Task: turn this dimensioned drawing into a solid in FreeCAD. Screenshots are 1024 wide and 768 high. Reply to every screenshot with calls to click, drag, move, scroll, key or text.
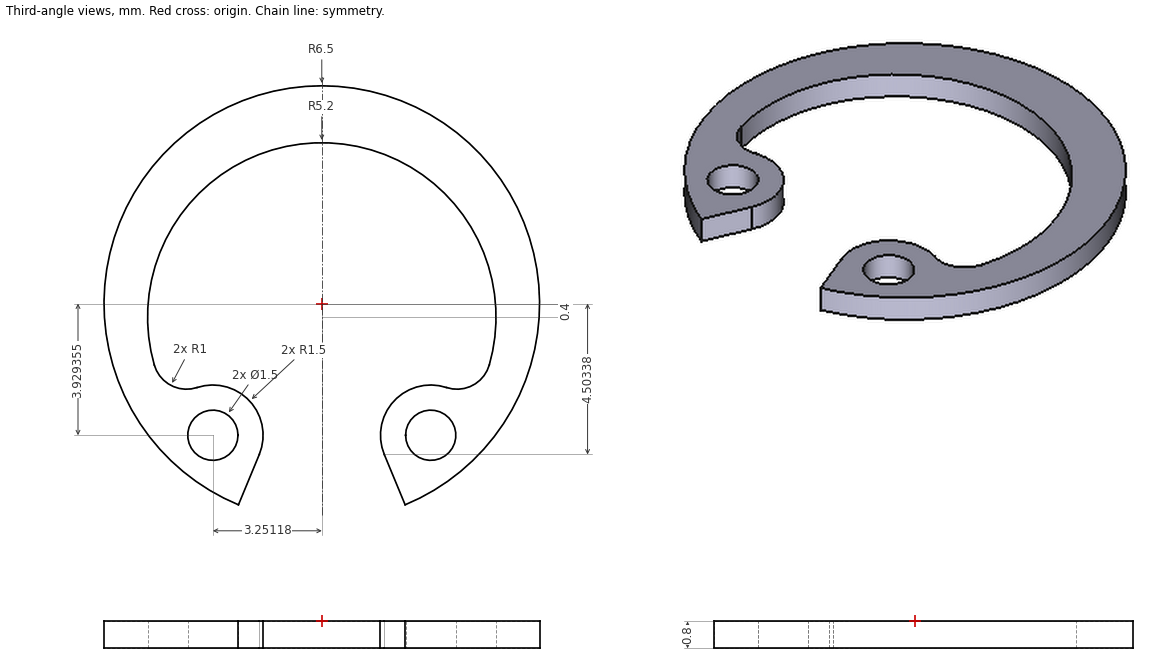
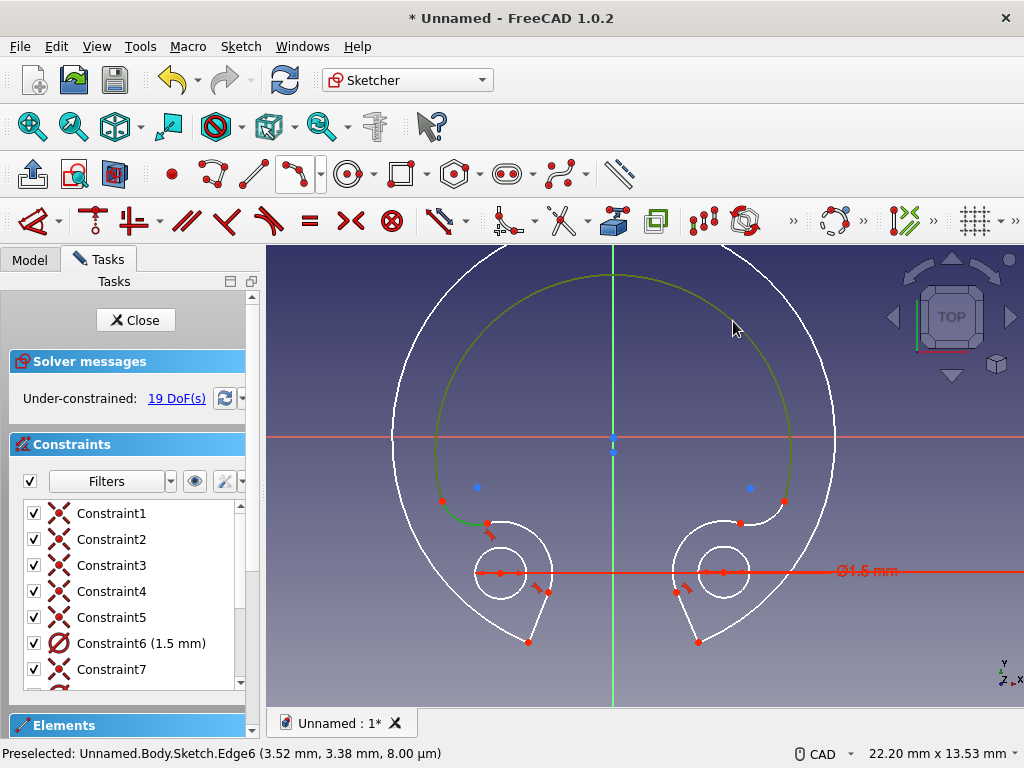
key(t)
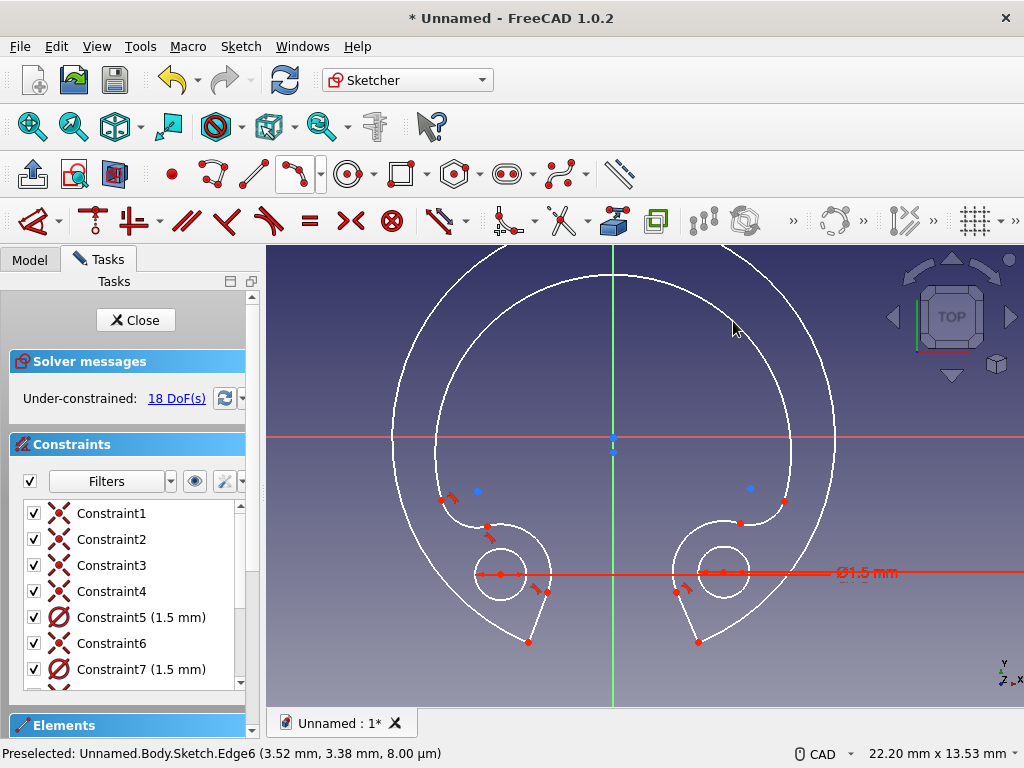
click(733, 321)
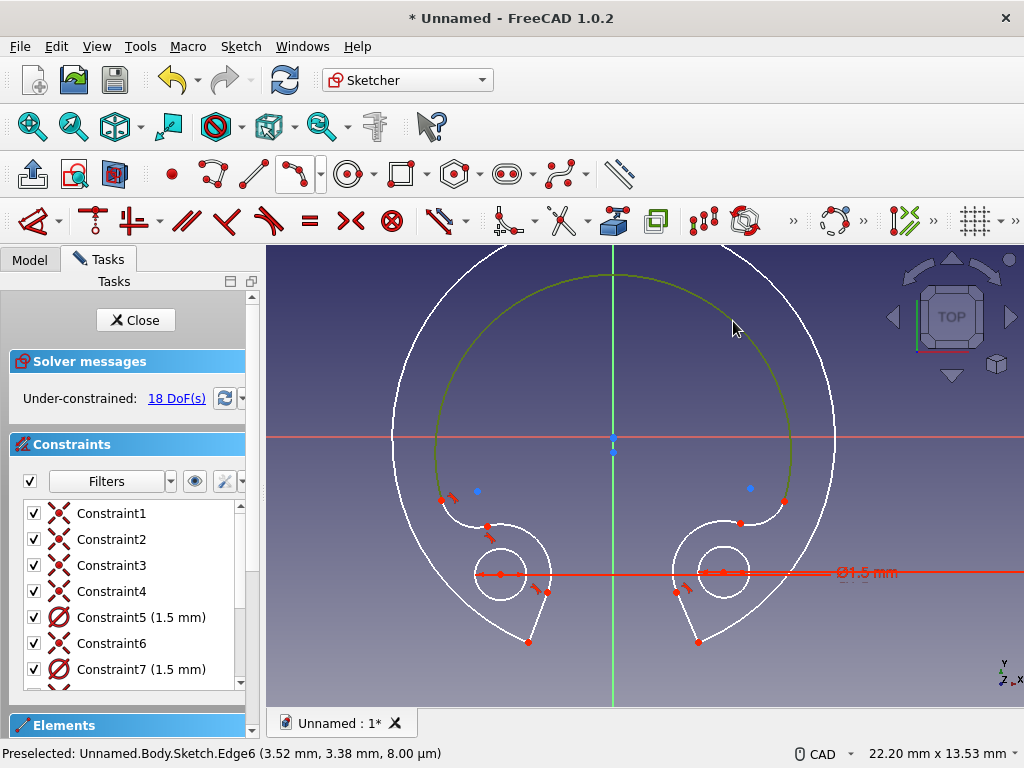
click(757, 524)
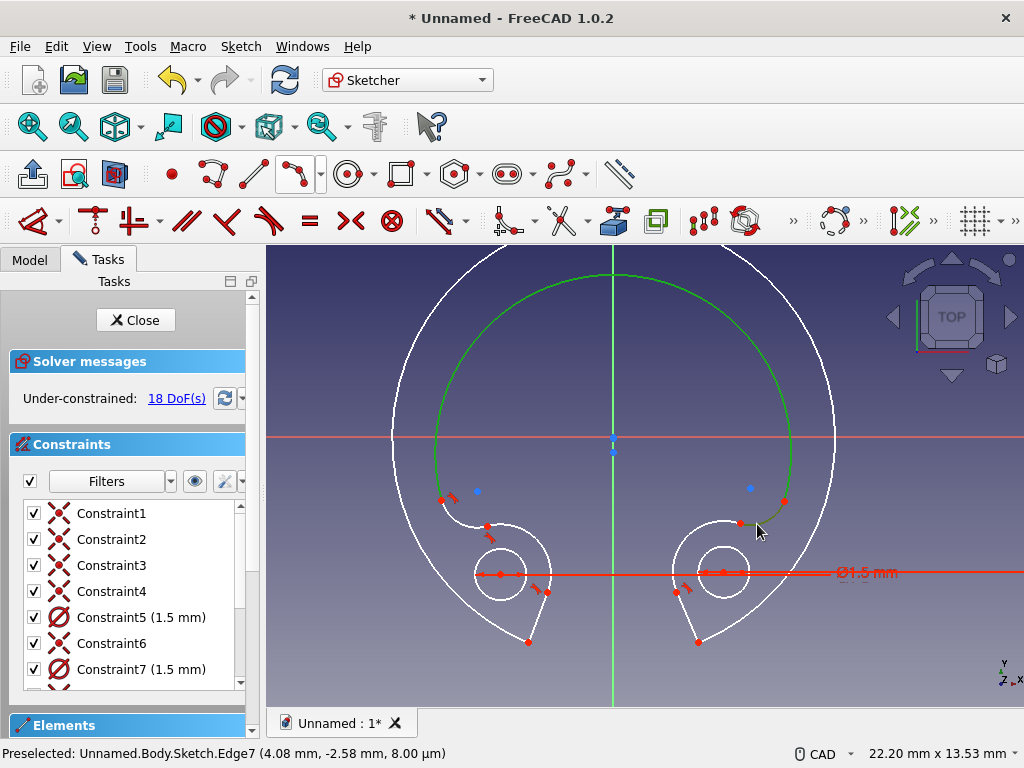
click(269, 222)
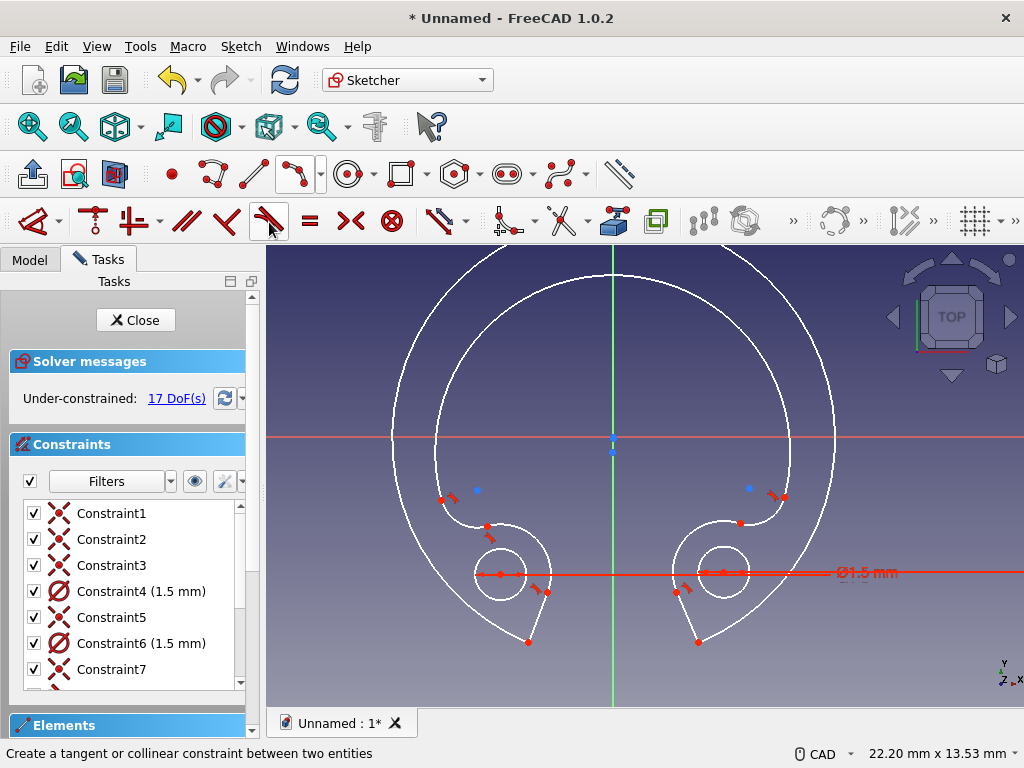
click(758, 524)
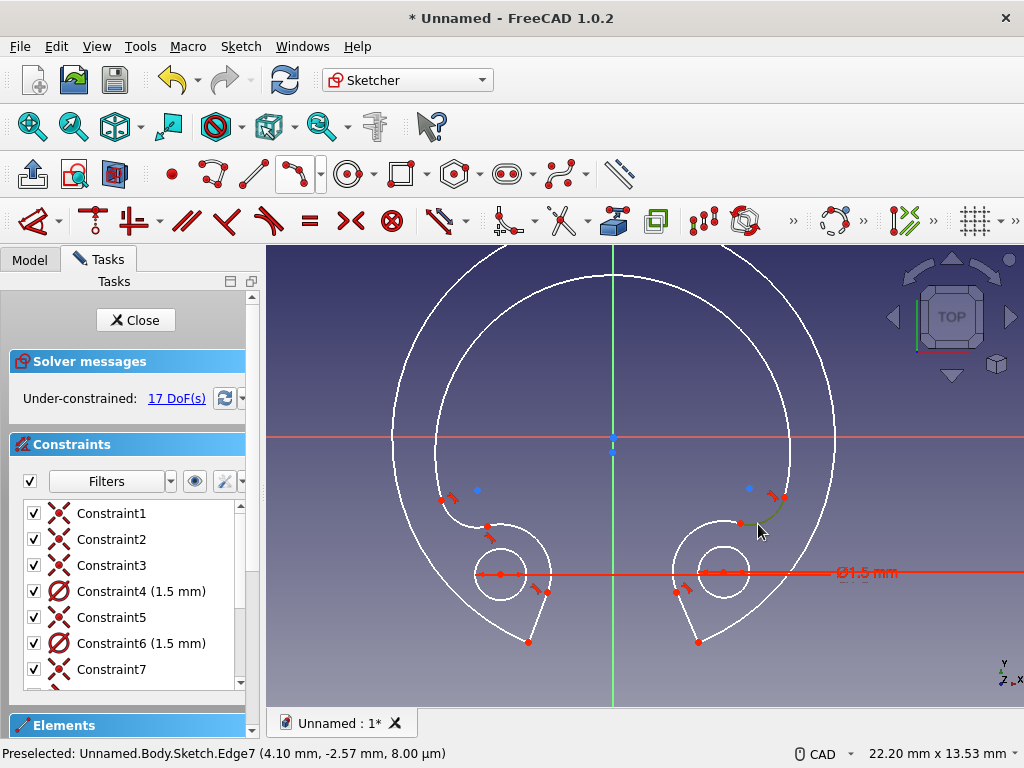
click(706, 524)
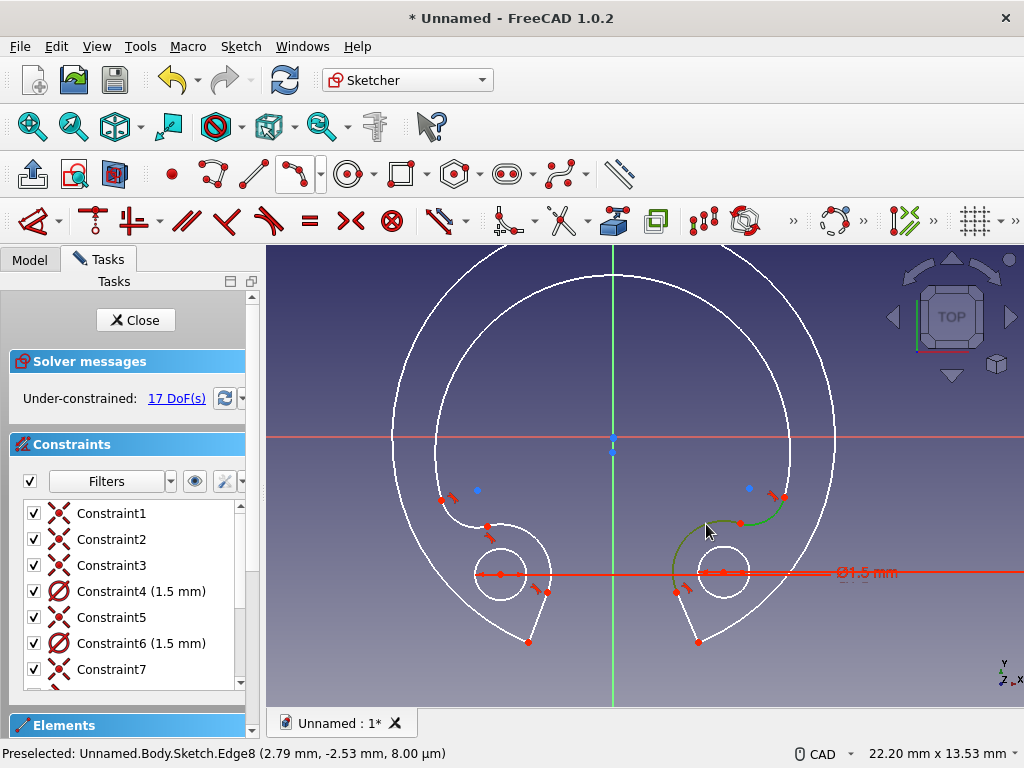
click(269, 222)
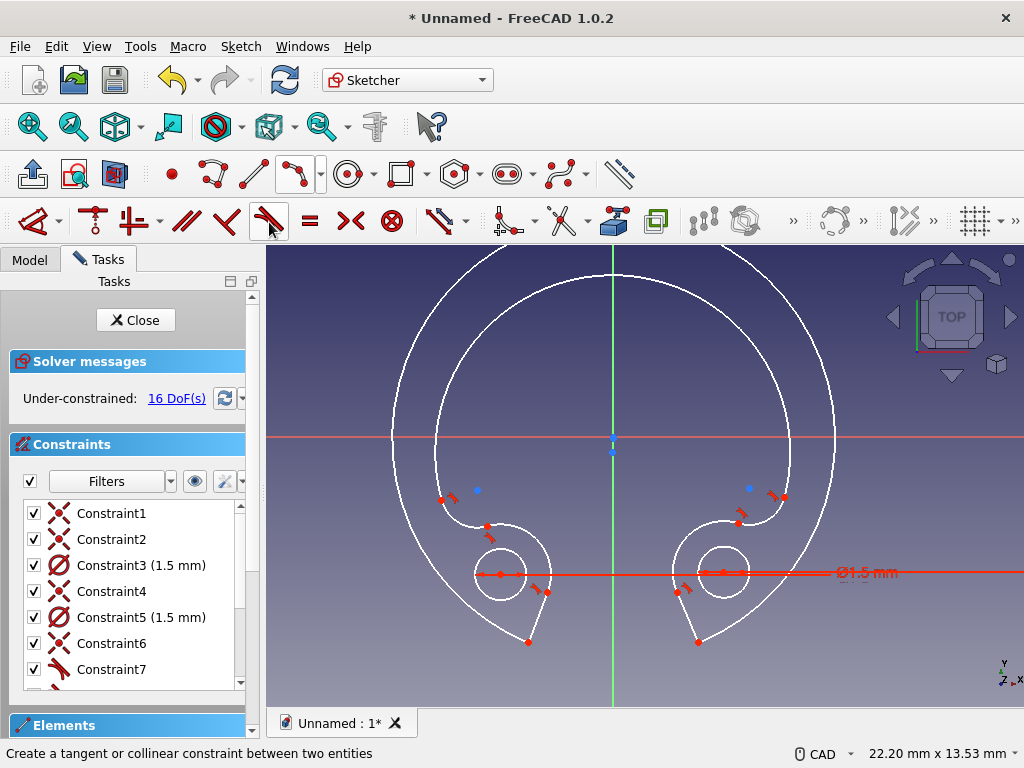
scroll(613, 438, up, 3)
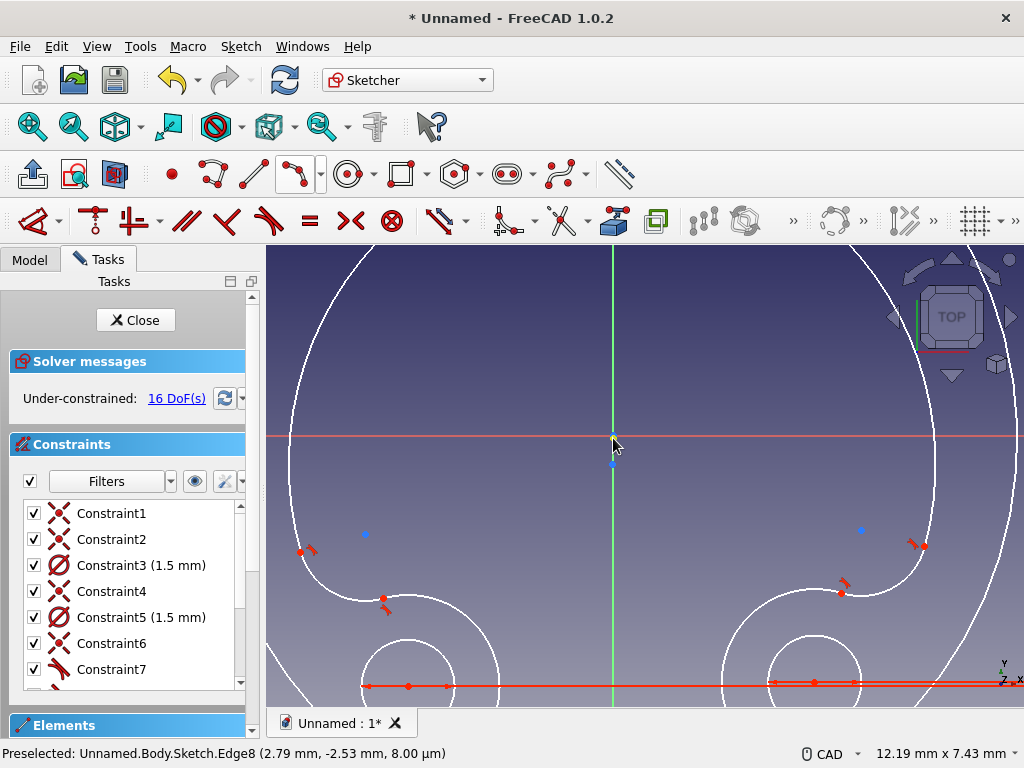
drag(603, 426, 624, 449)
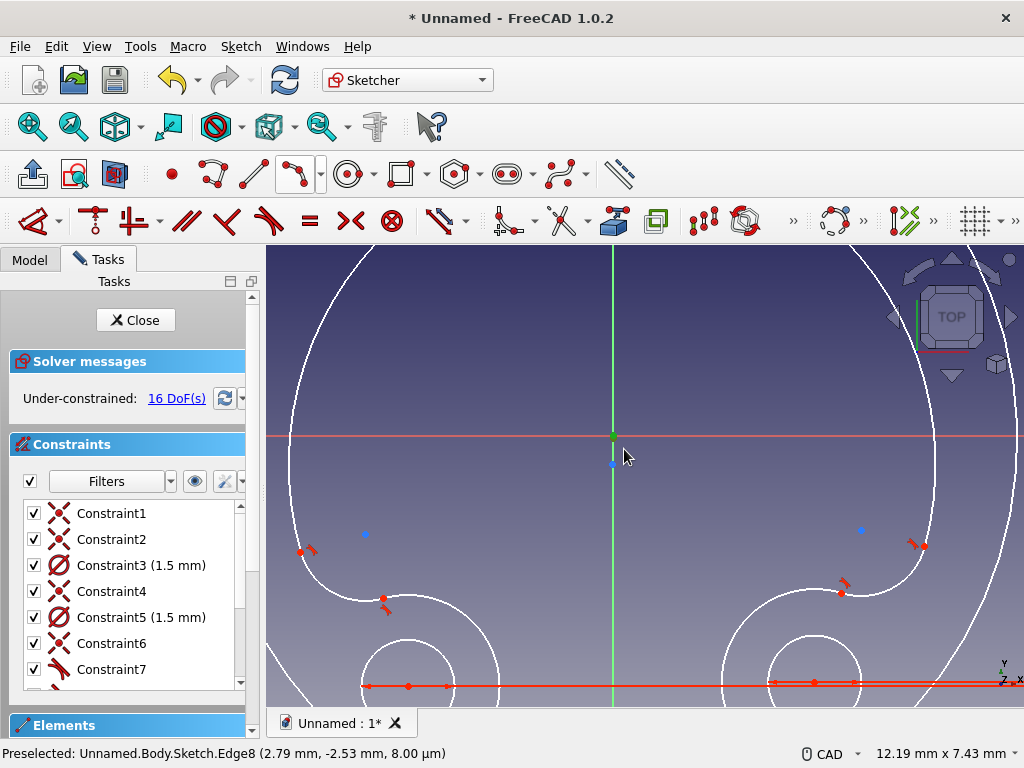
click(93, 222)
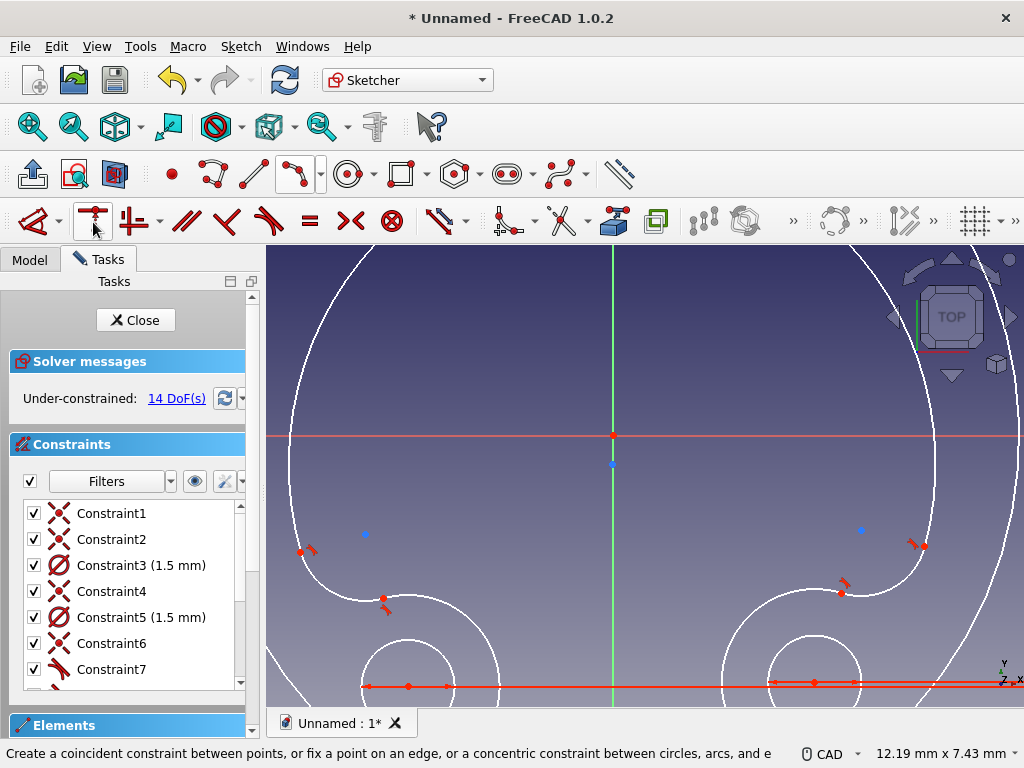
click(316, 579)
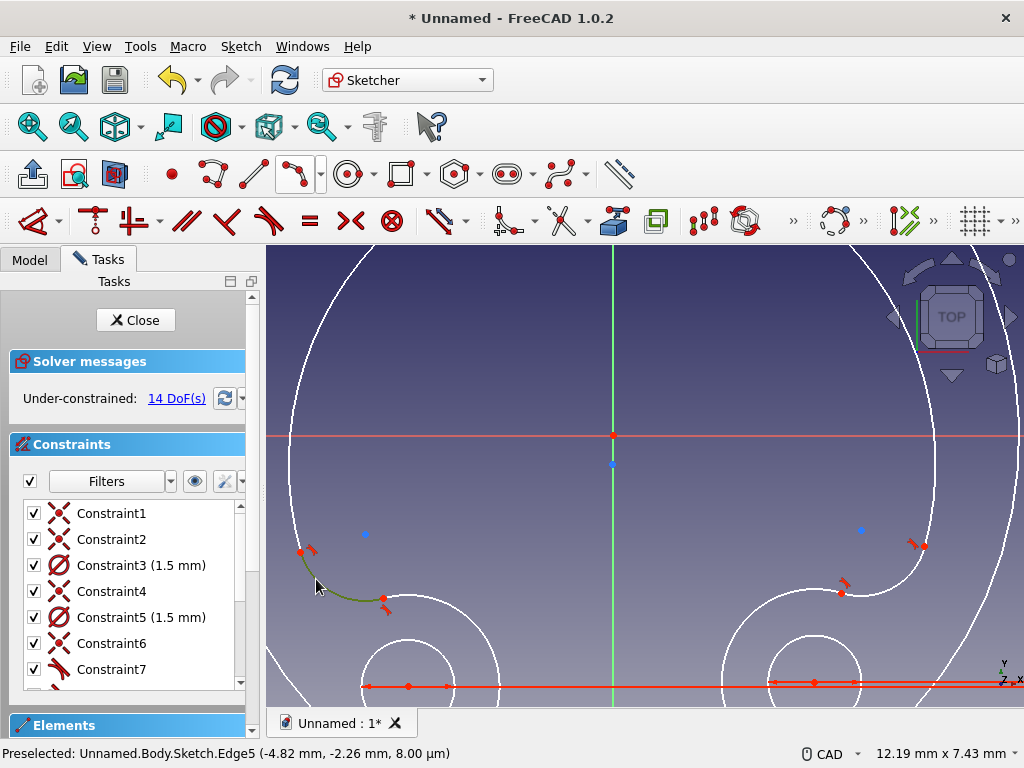
scroll(555, 508, down, 5)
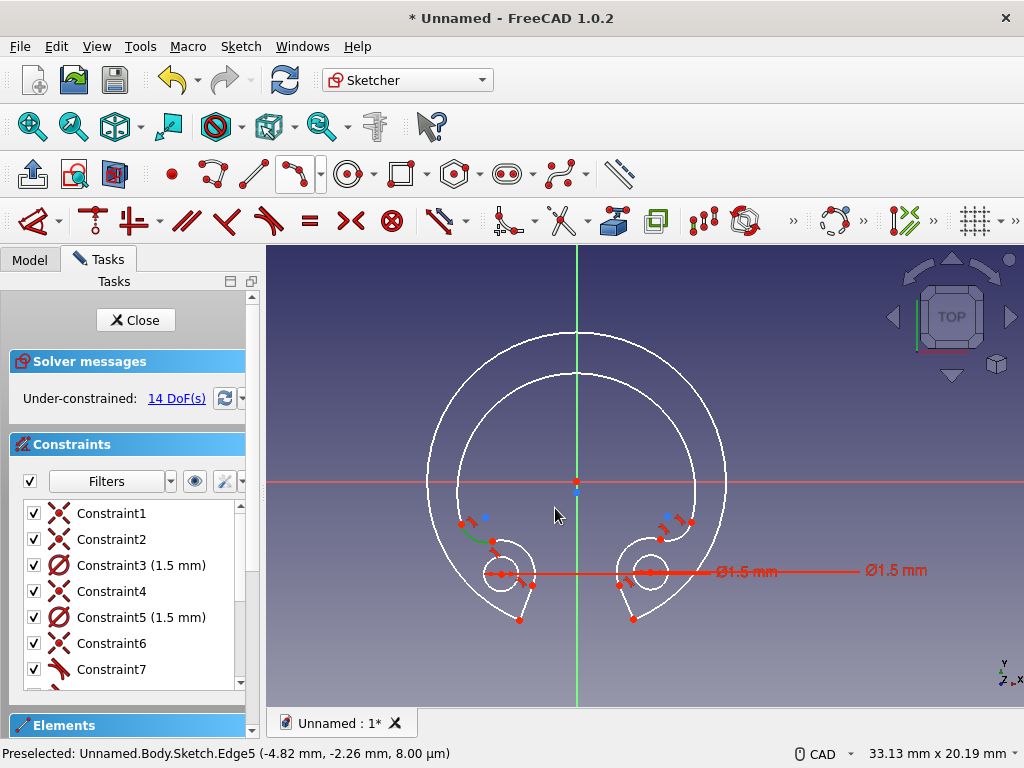
click(672, 540)